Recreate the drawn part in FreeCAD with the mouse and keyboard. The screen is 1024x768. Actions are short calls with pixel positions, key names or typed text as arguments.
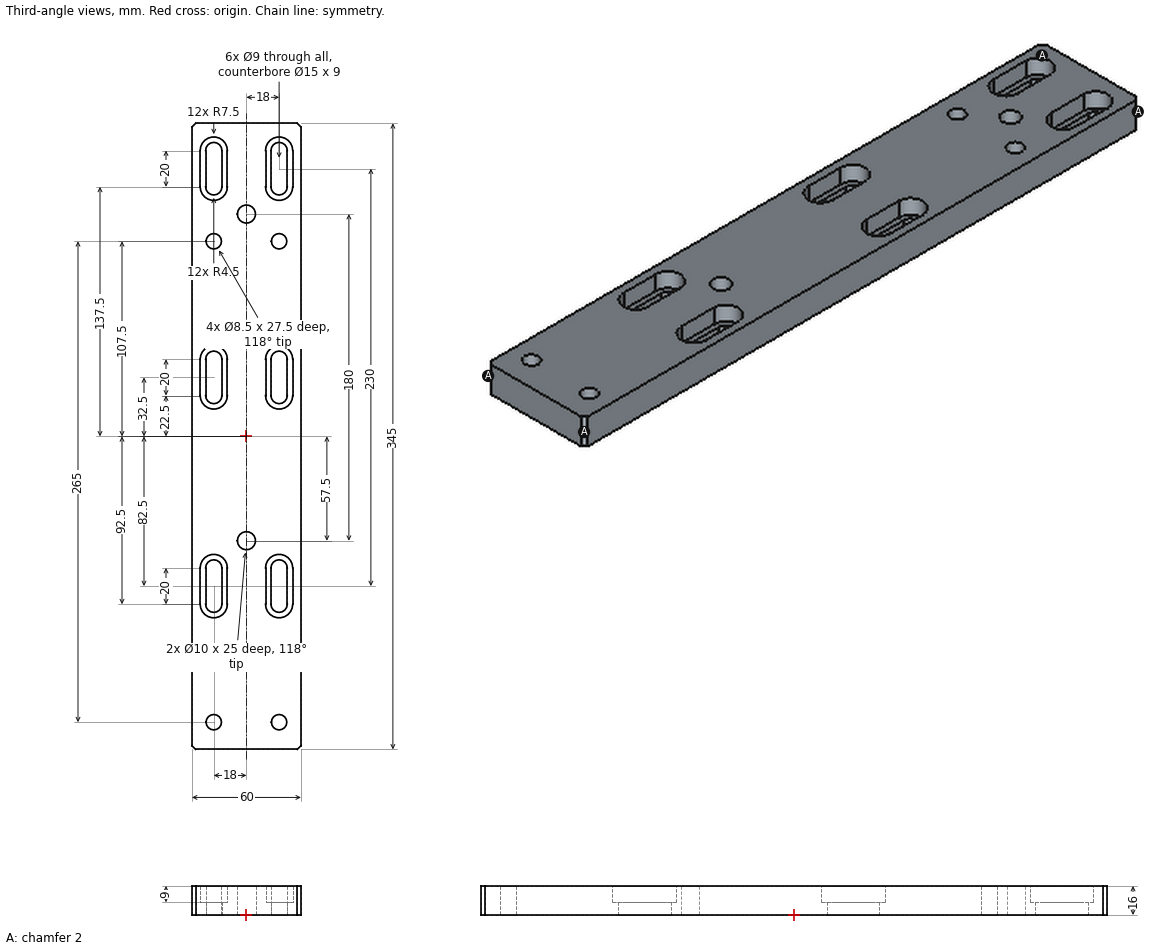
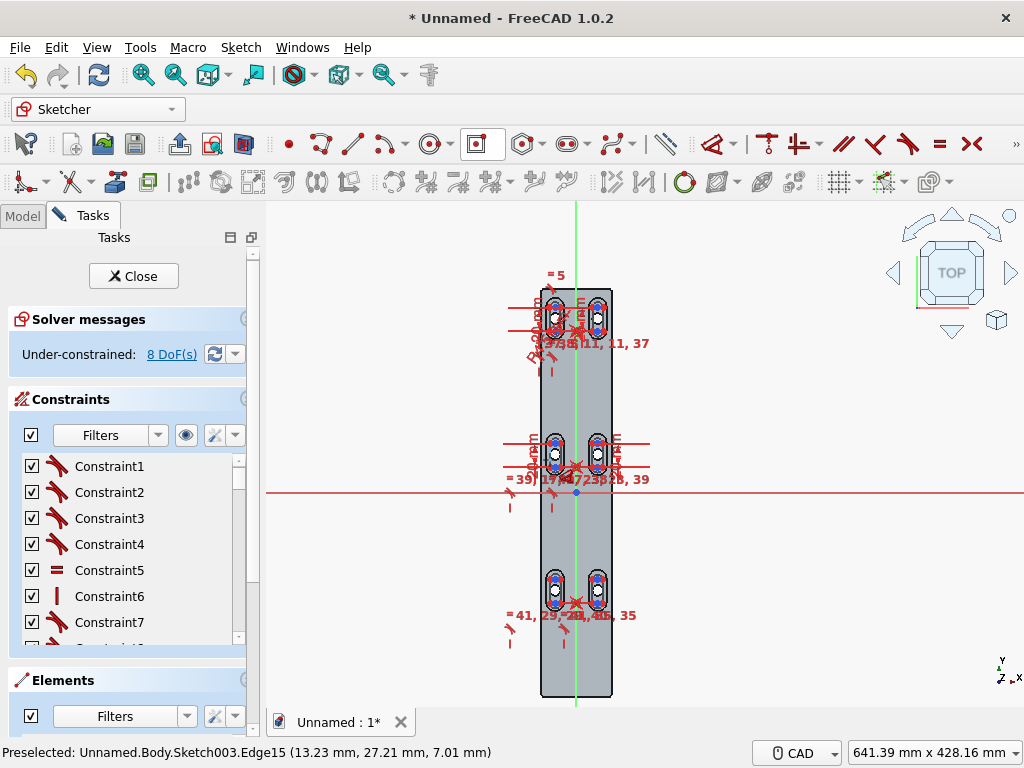
scroll(550, 596, up, 4)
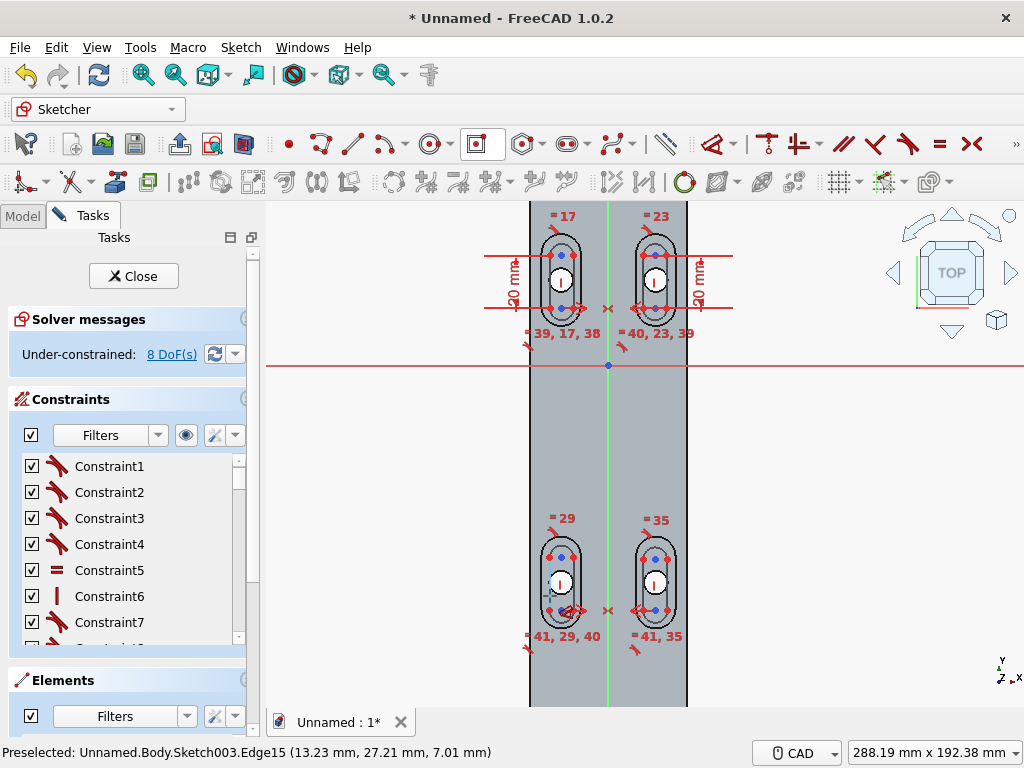
click(550, 595)
click(516, 584)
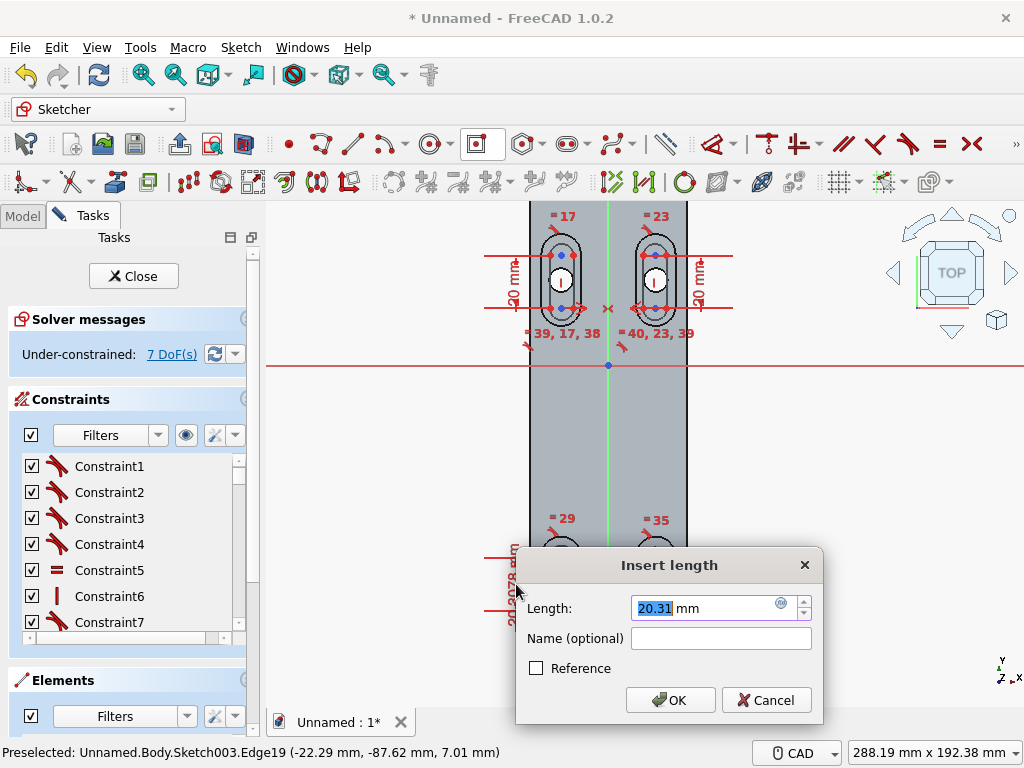
text(20)
key(Return)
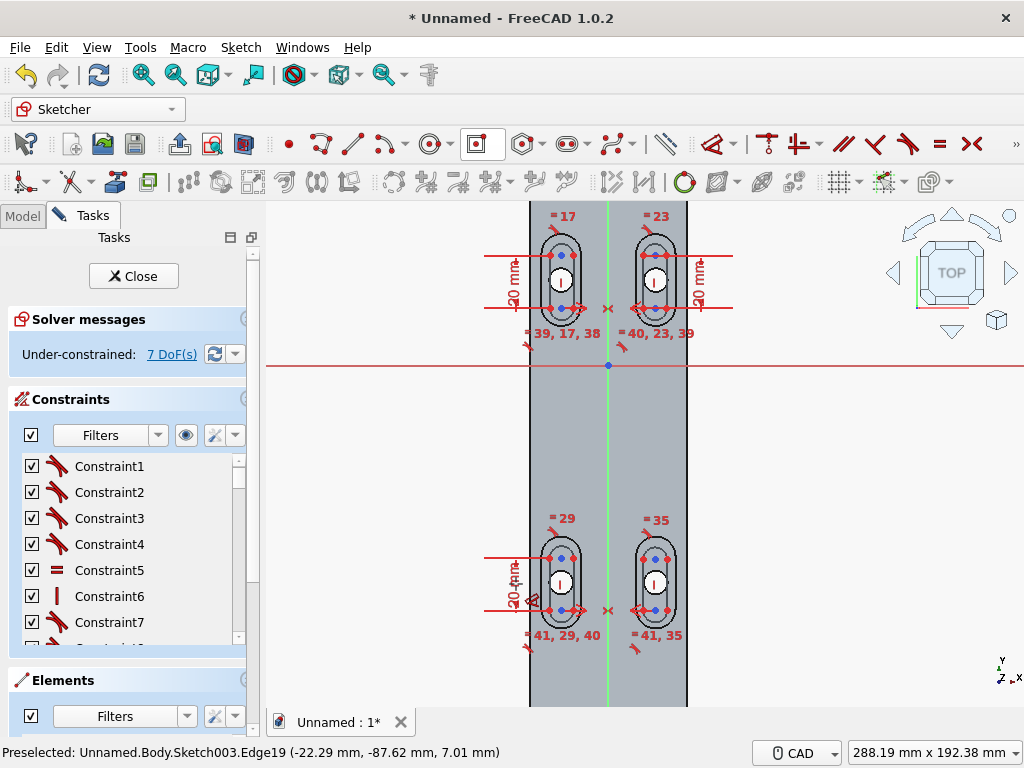
click(643, 595)
click(701, 585)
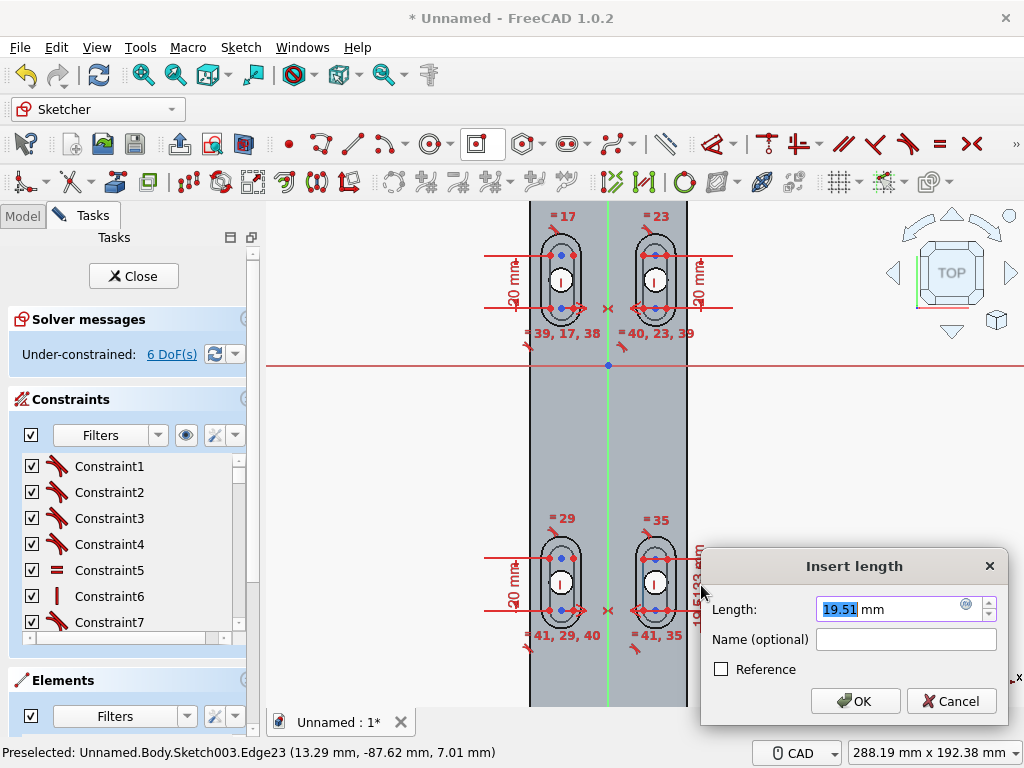
text(20)
key(Return)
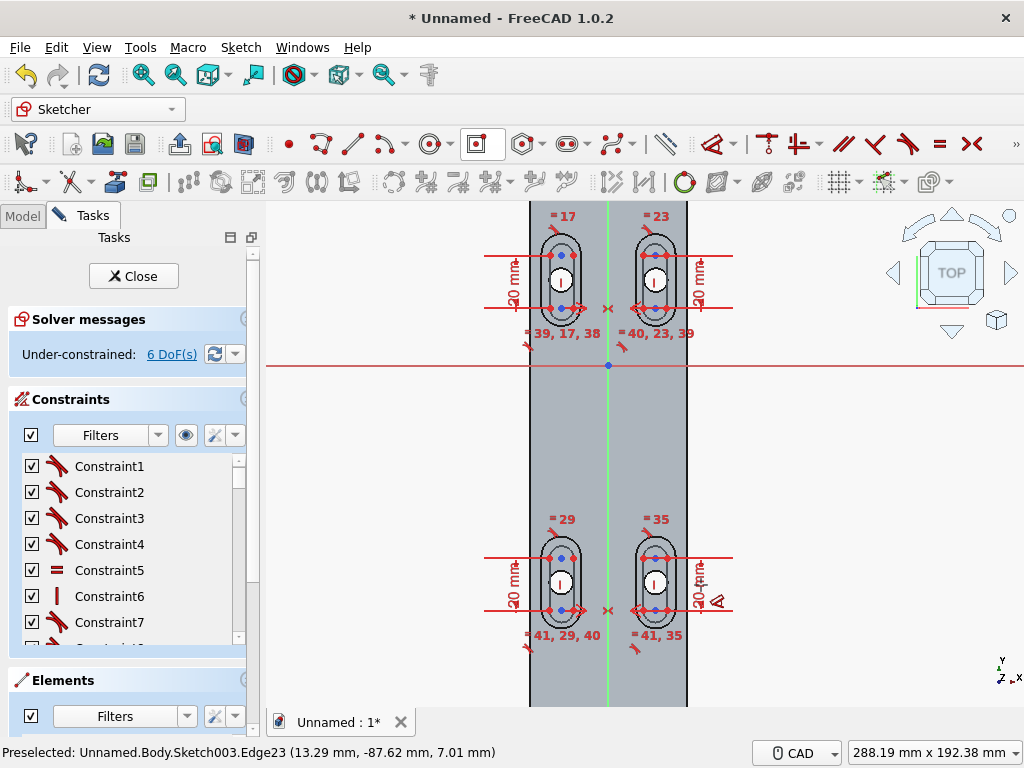
scroll(550, 596, down, 4)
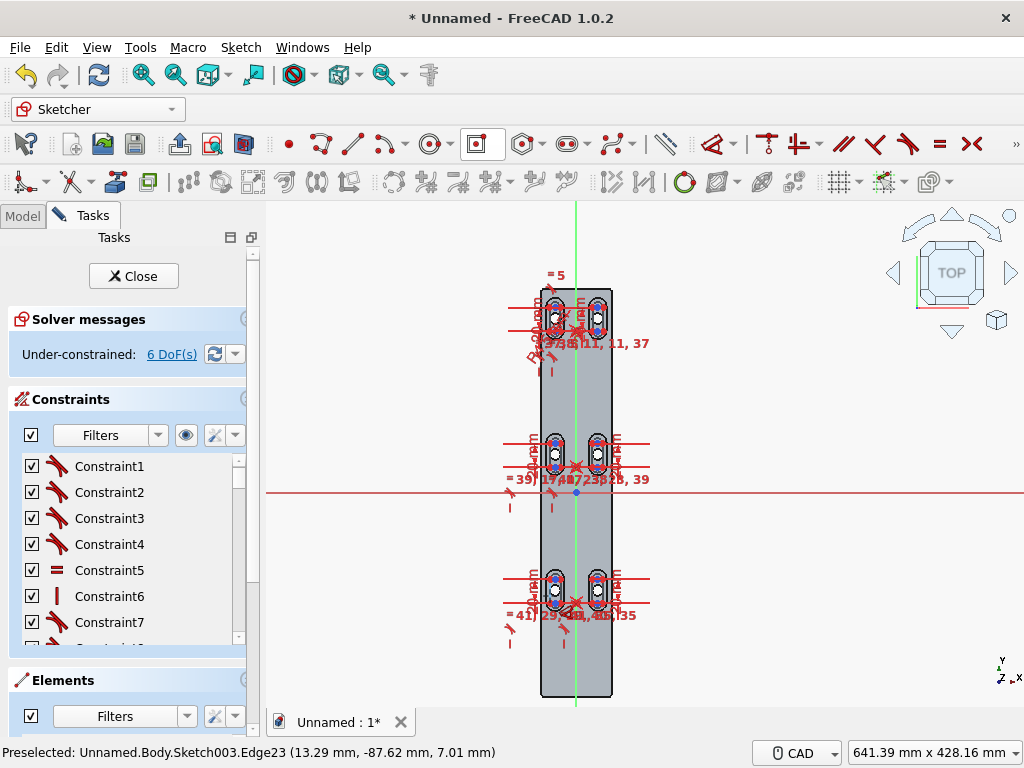
scroll(555, 331, up, 5)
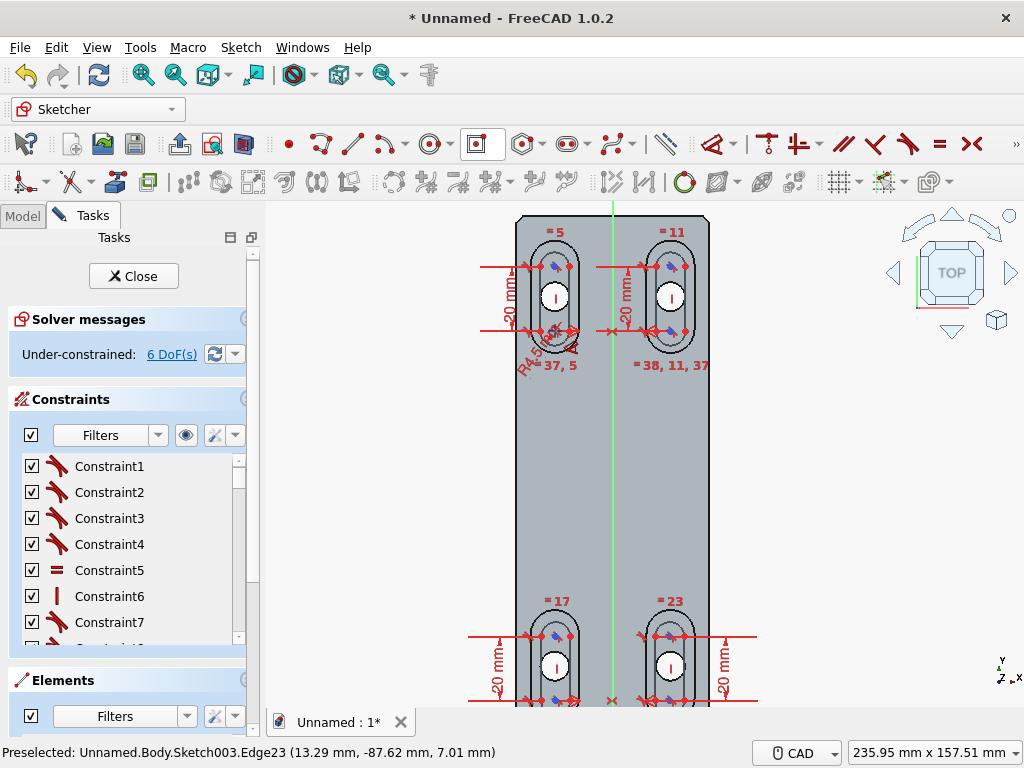
click(555, 331)
click(584, 273)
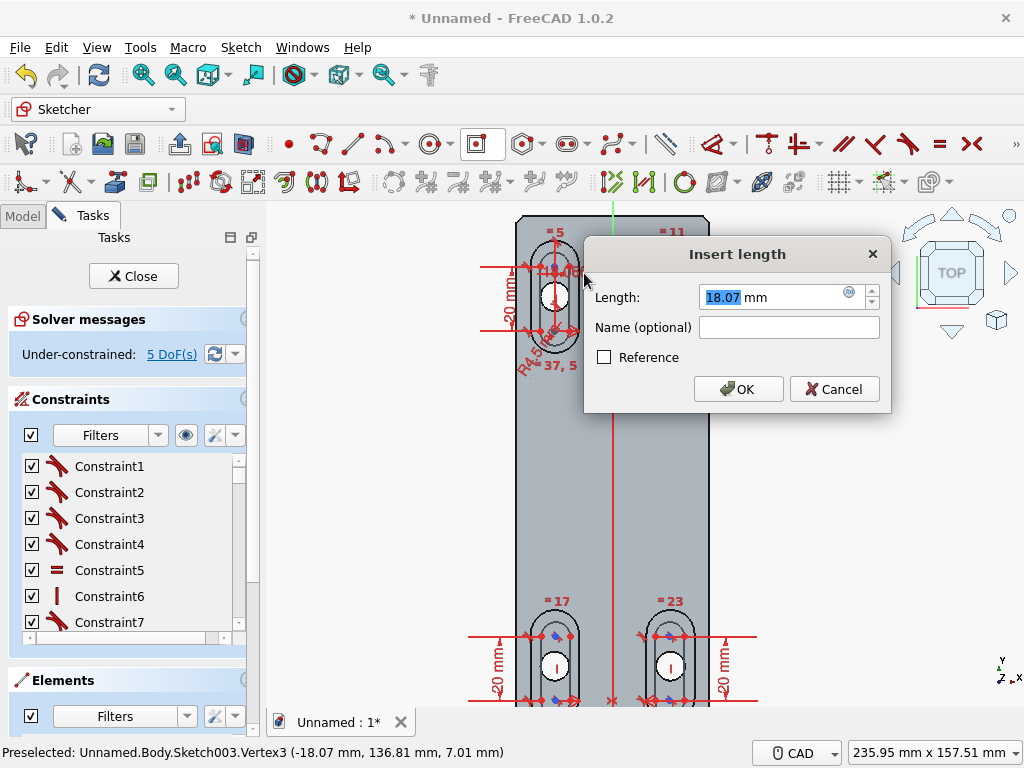
text(18)
key(Return)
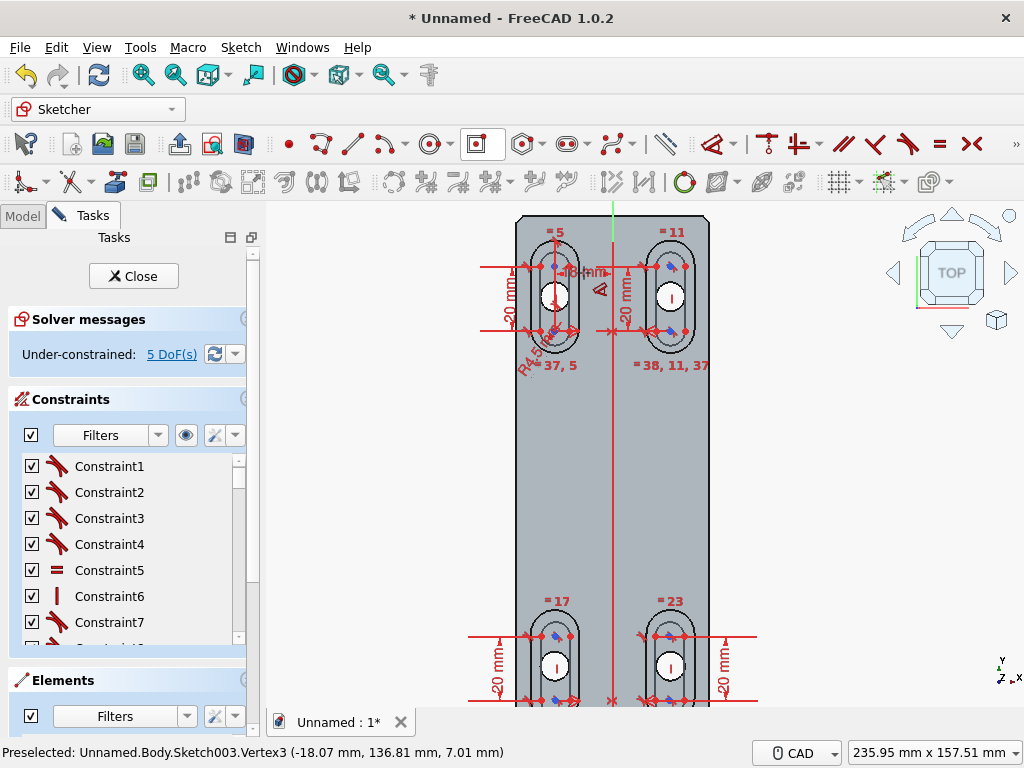
scroll(555, 331, down, 5)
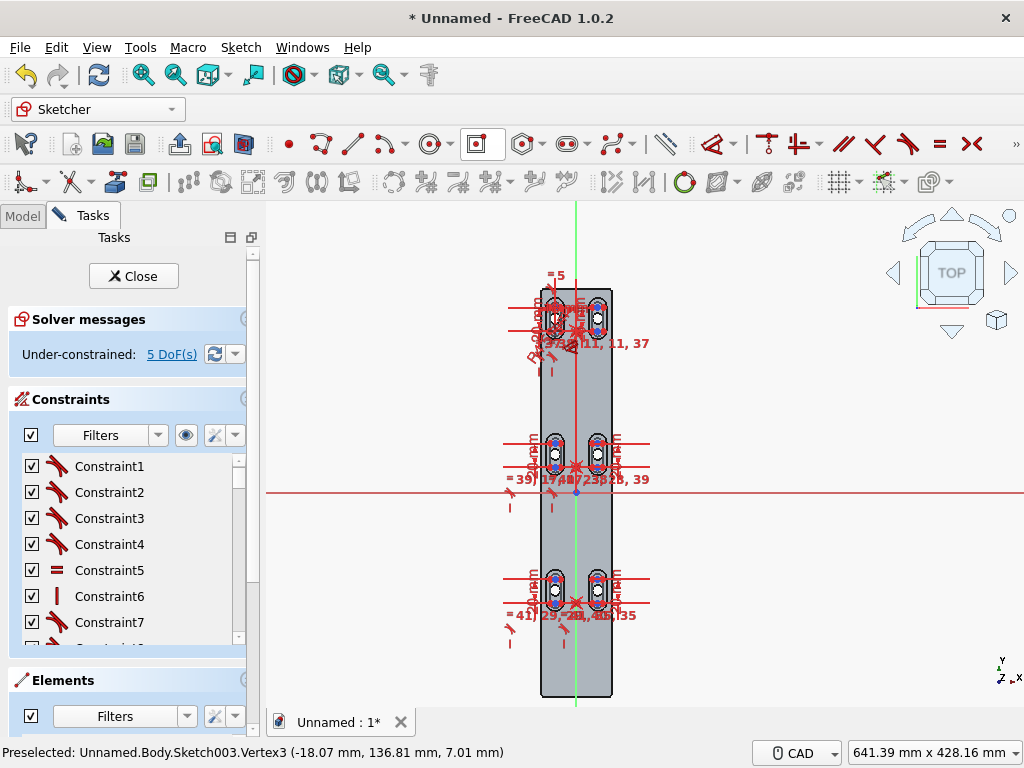
scroll(556, 467, up, 5)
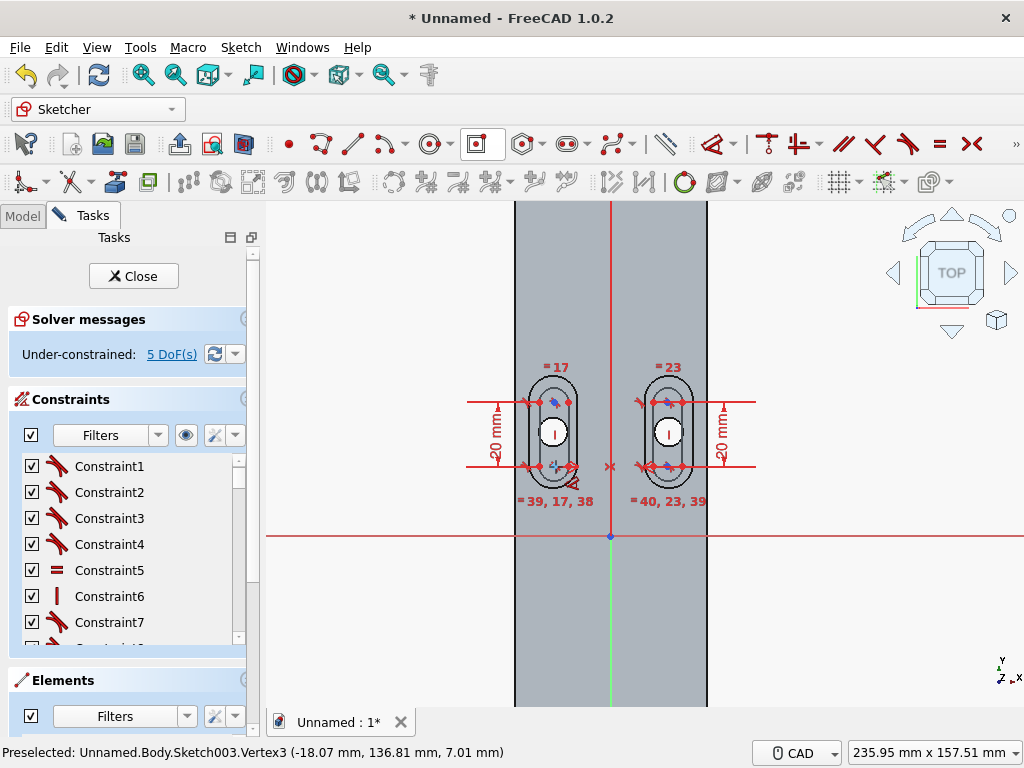
click(554, 467)
click(583, 570)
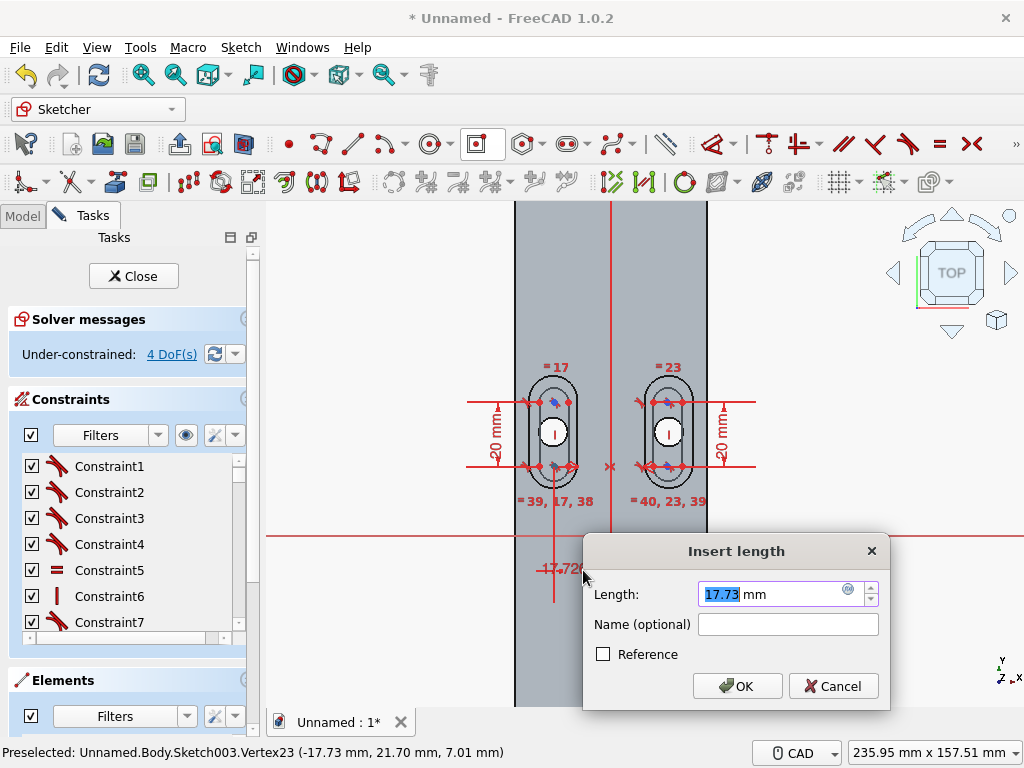
text(18)
key(Return)